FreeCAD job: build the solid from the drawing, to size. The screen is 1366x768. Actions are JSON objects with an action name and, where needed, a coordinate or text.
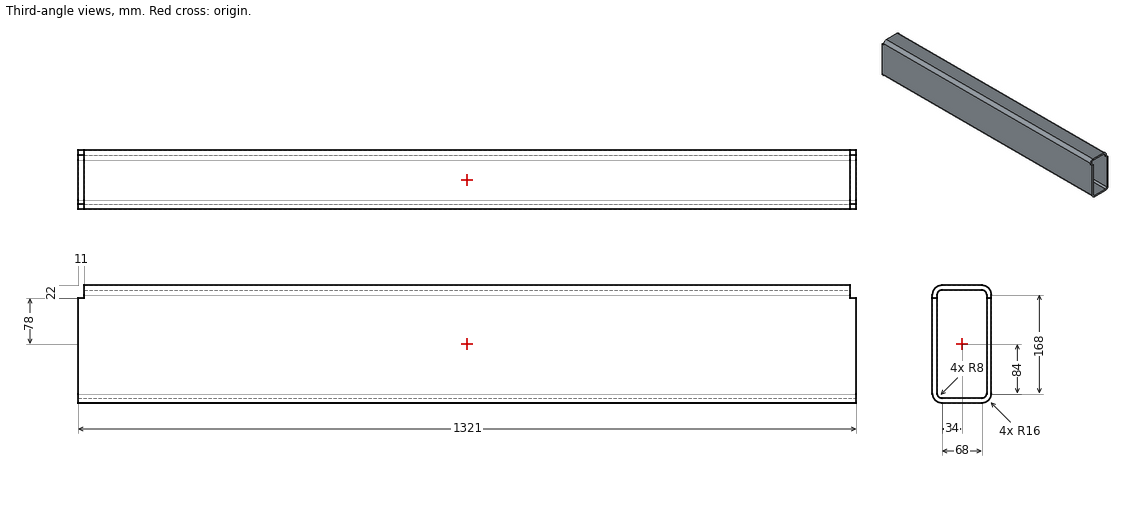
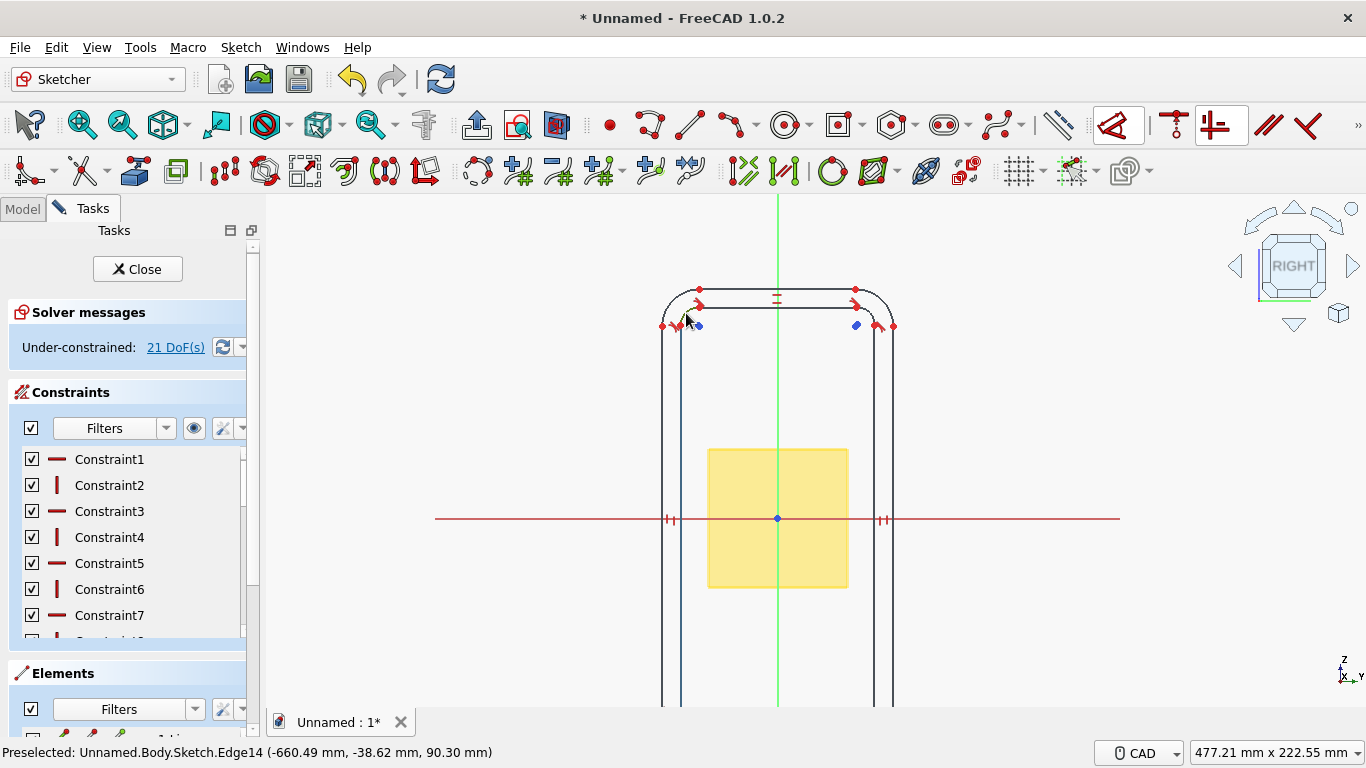
{"action": "key", "text": "t"}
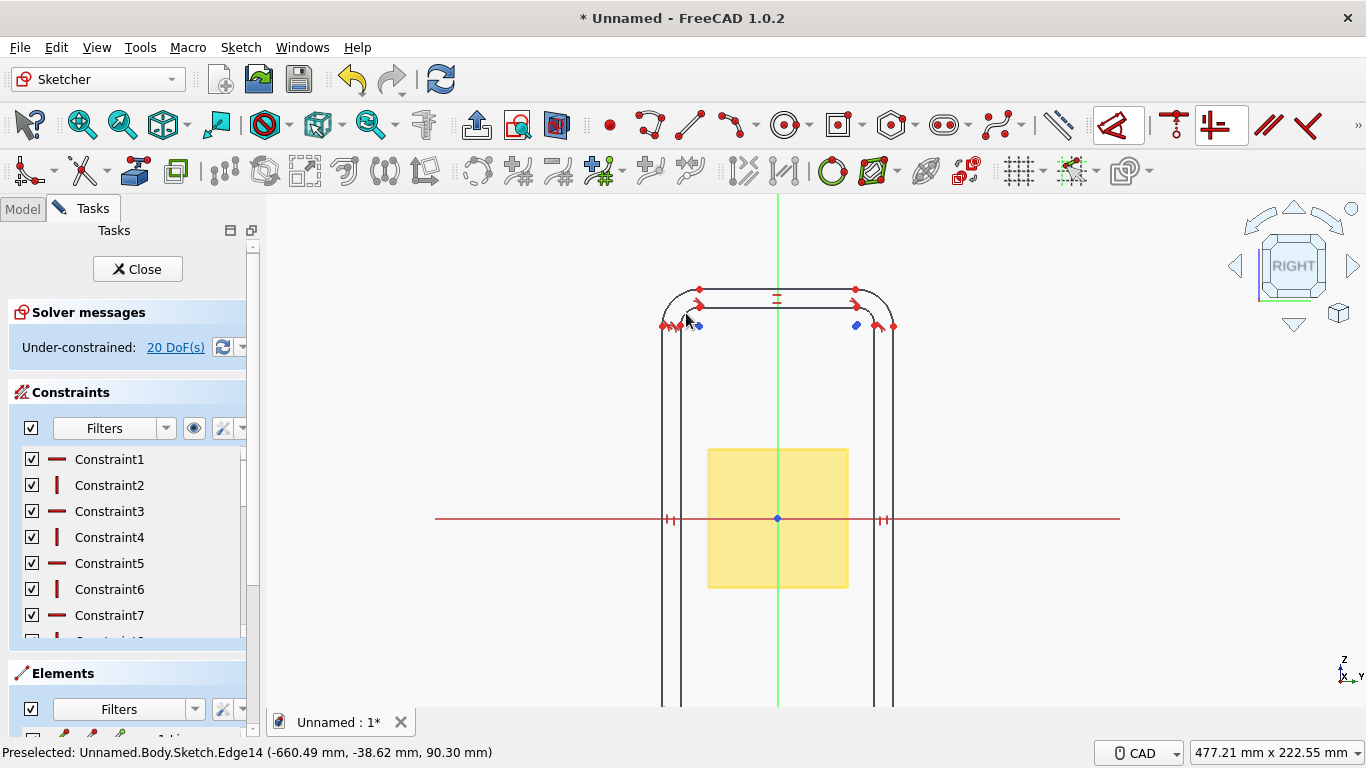
{"action": "left_click", "coordinate": [746, 308]}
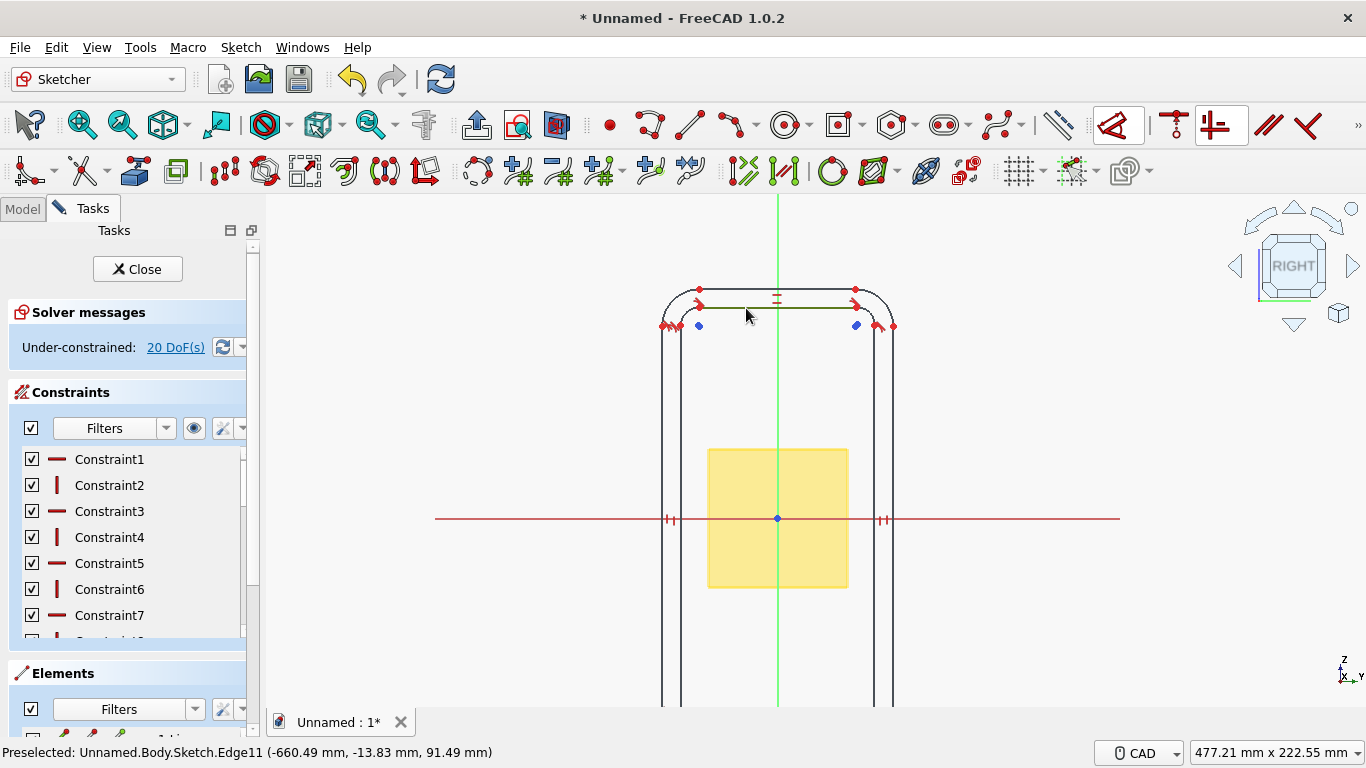
{"action": "left_click", "coordinate": [686, 313]}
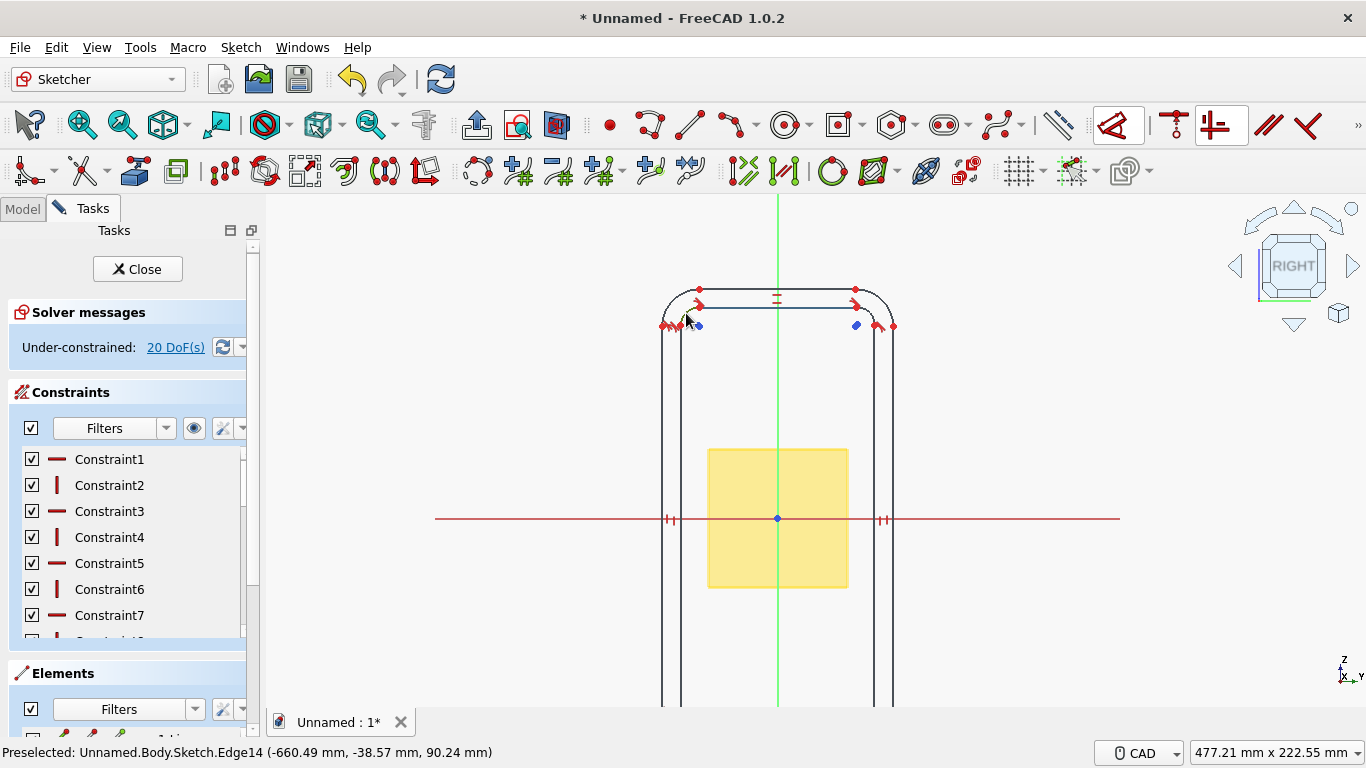
{"action": "key", "text": "t"}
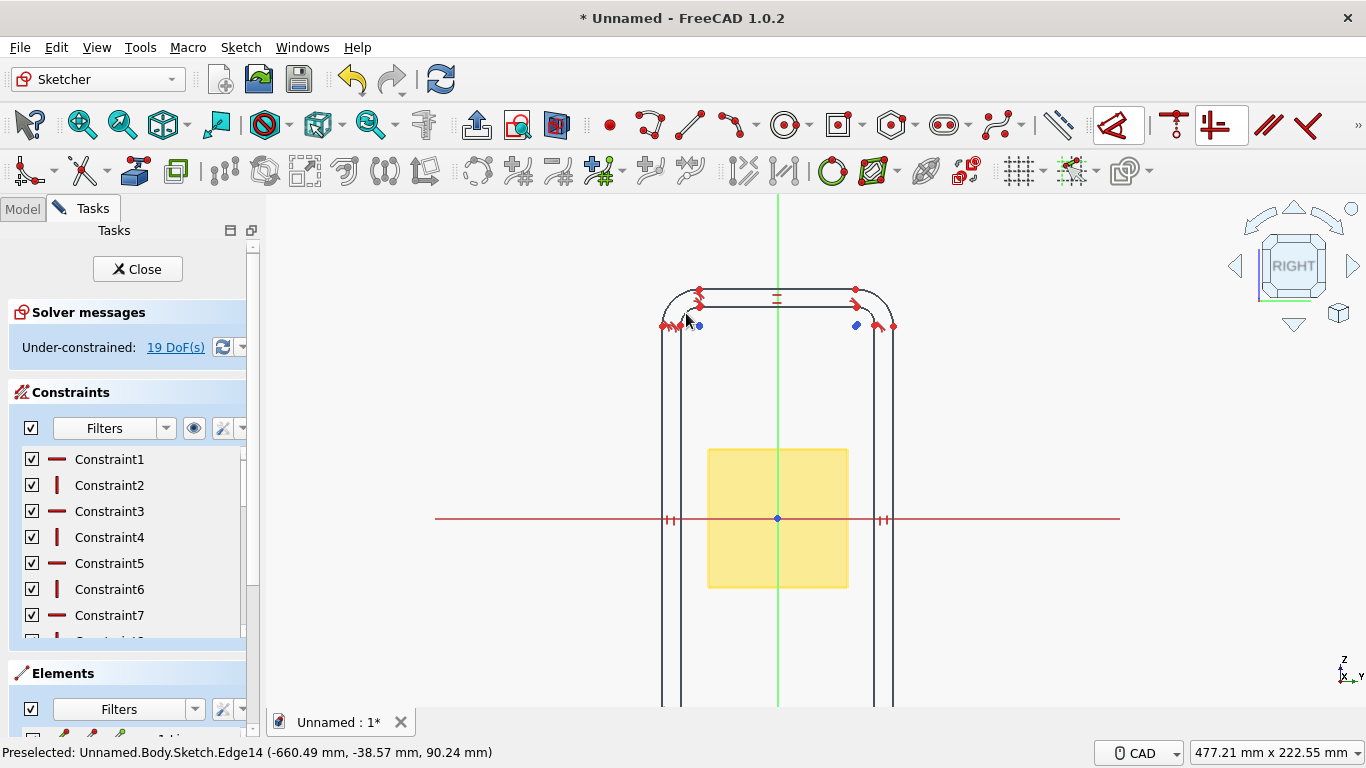
{"action": "left_click", "coordinate": [746, 307]}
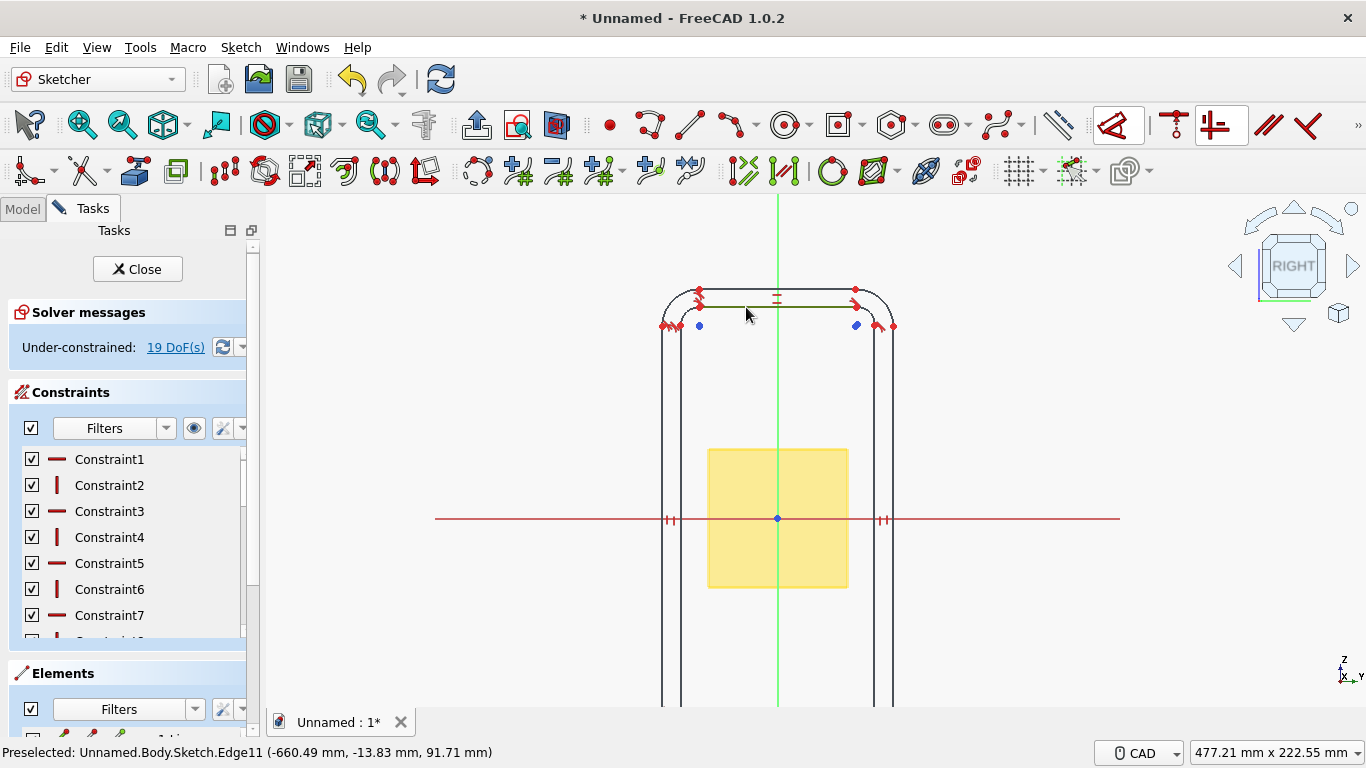
{"action": "left_click", "coordinate": [870, 312]}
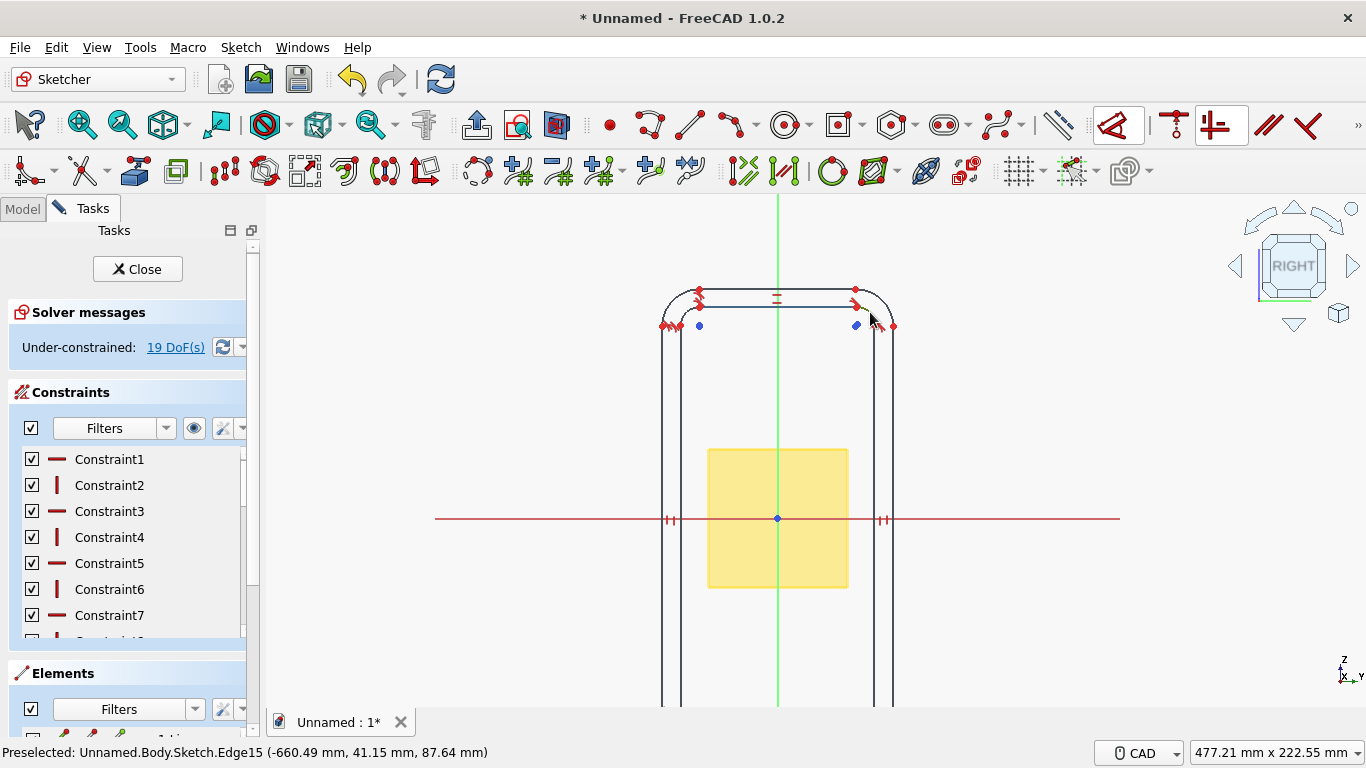
{"action": "key", "text": "t"}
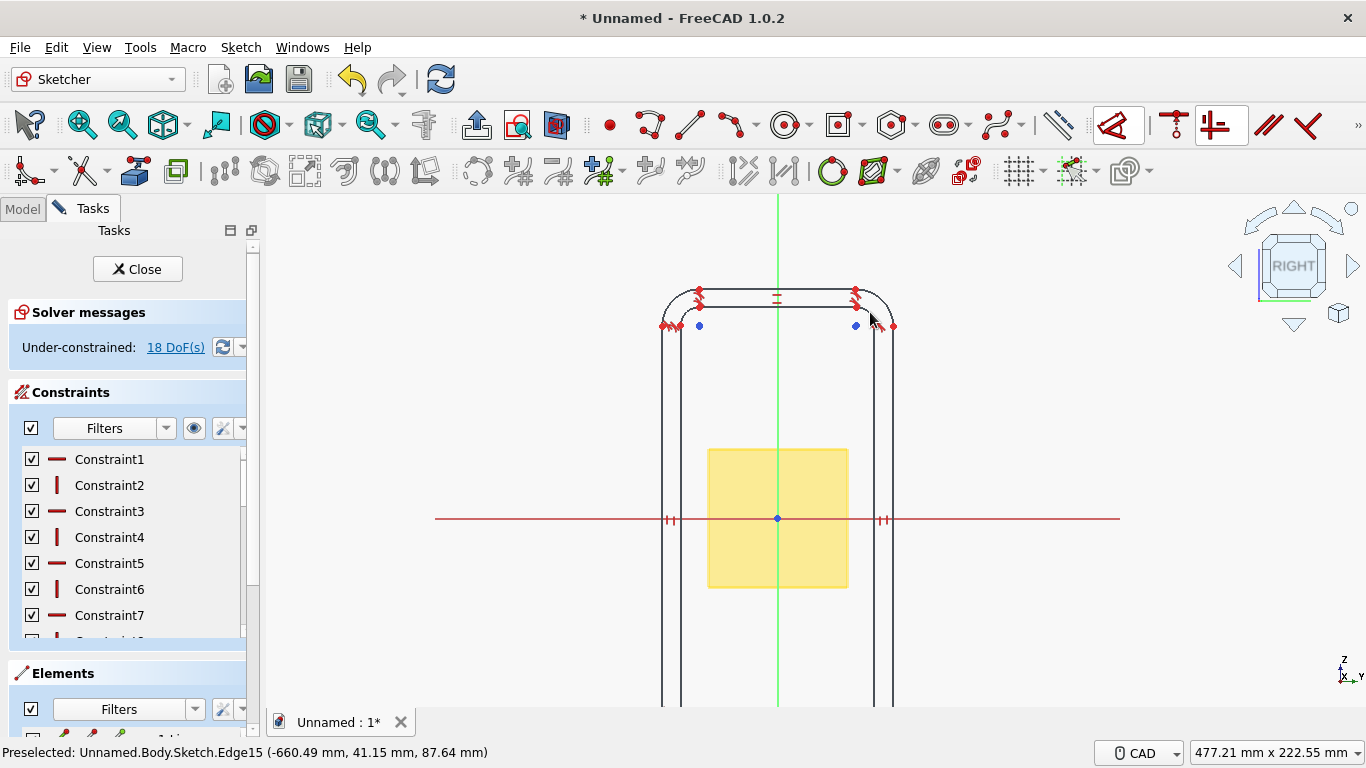
{"action": "left_click", "coordinate": [874, 442]}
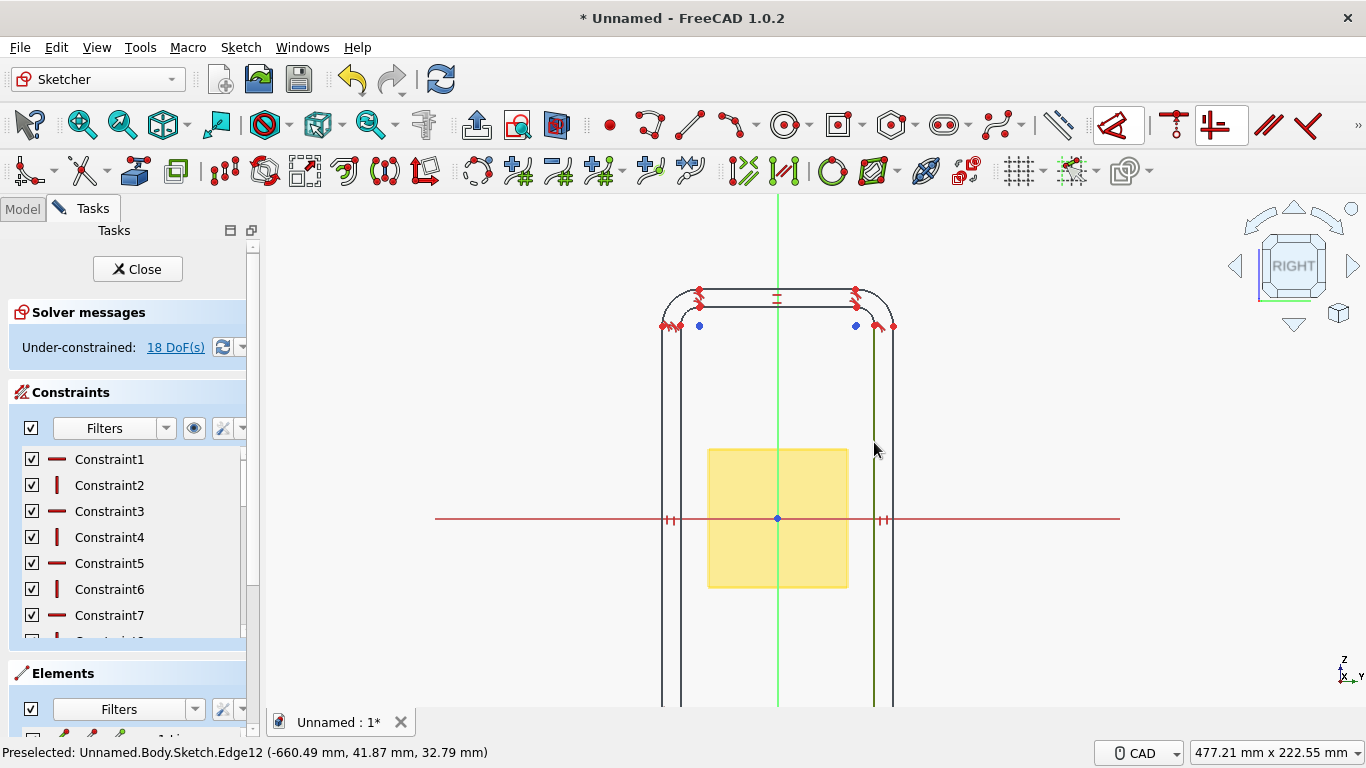
{"action": "left_click", "coordinate": [869, 313]}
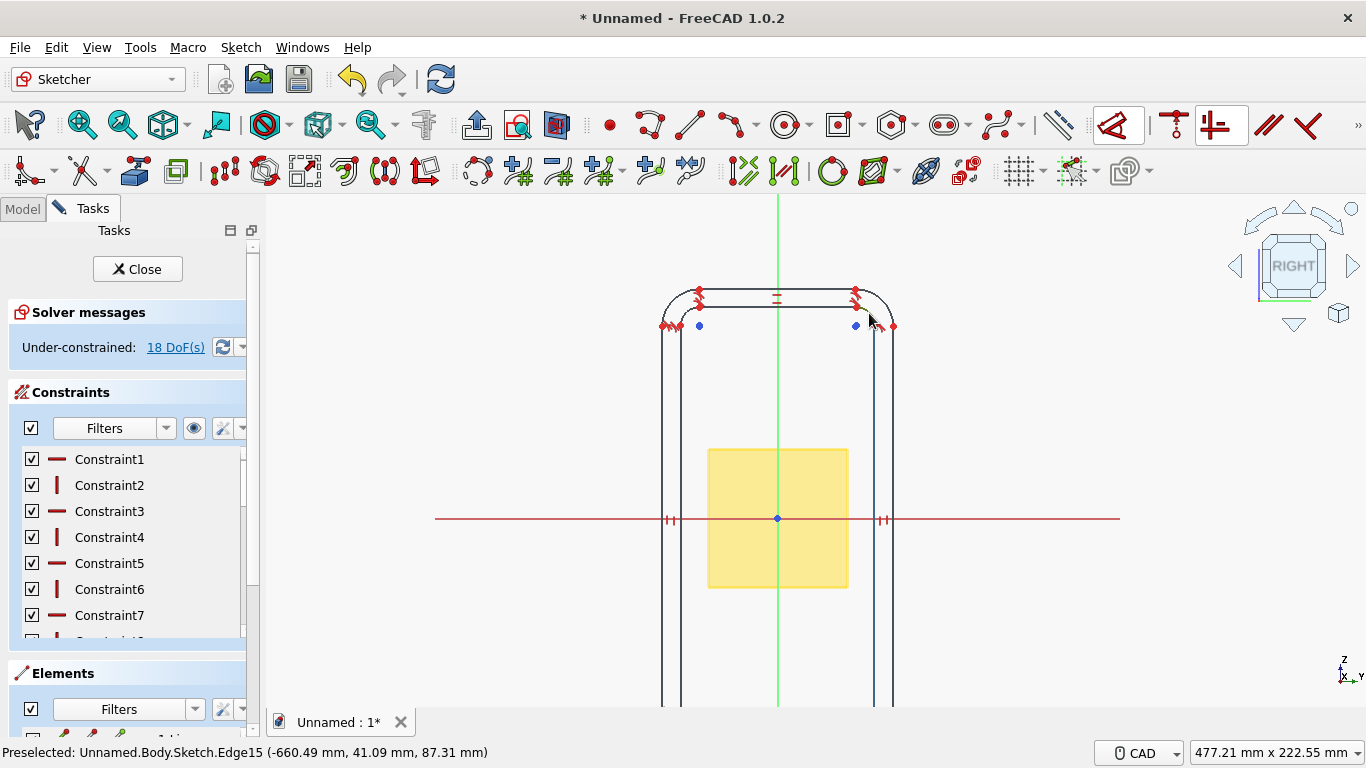
{"action": "key", "text": "t"}